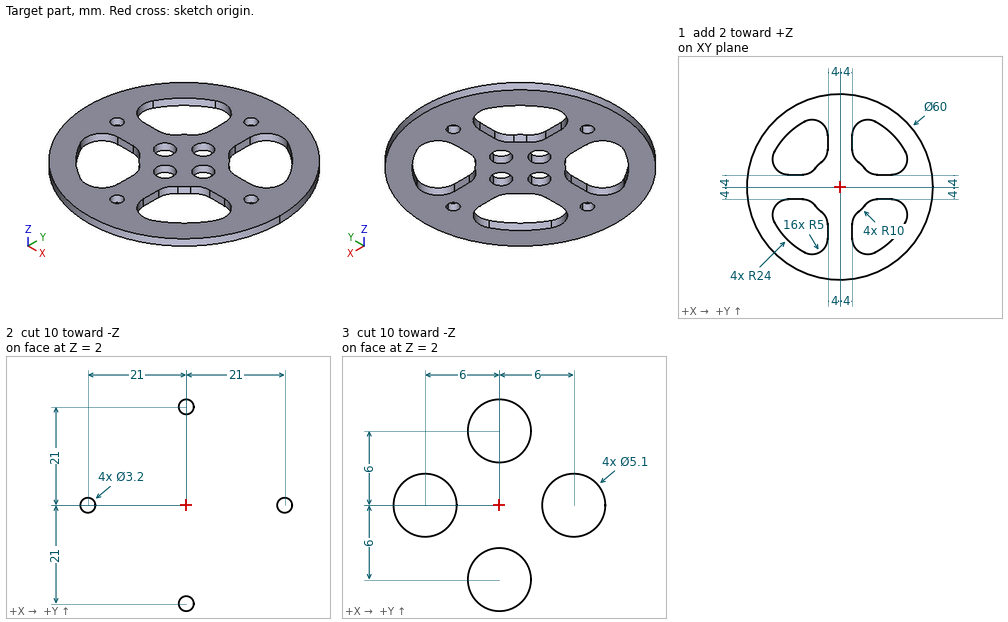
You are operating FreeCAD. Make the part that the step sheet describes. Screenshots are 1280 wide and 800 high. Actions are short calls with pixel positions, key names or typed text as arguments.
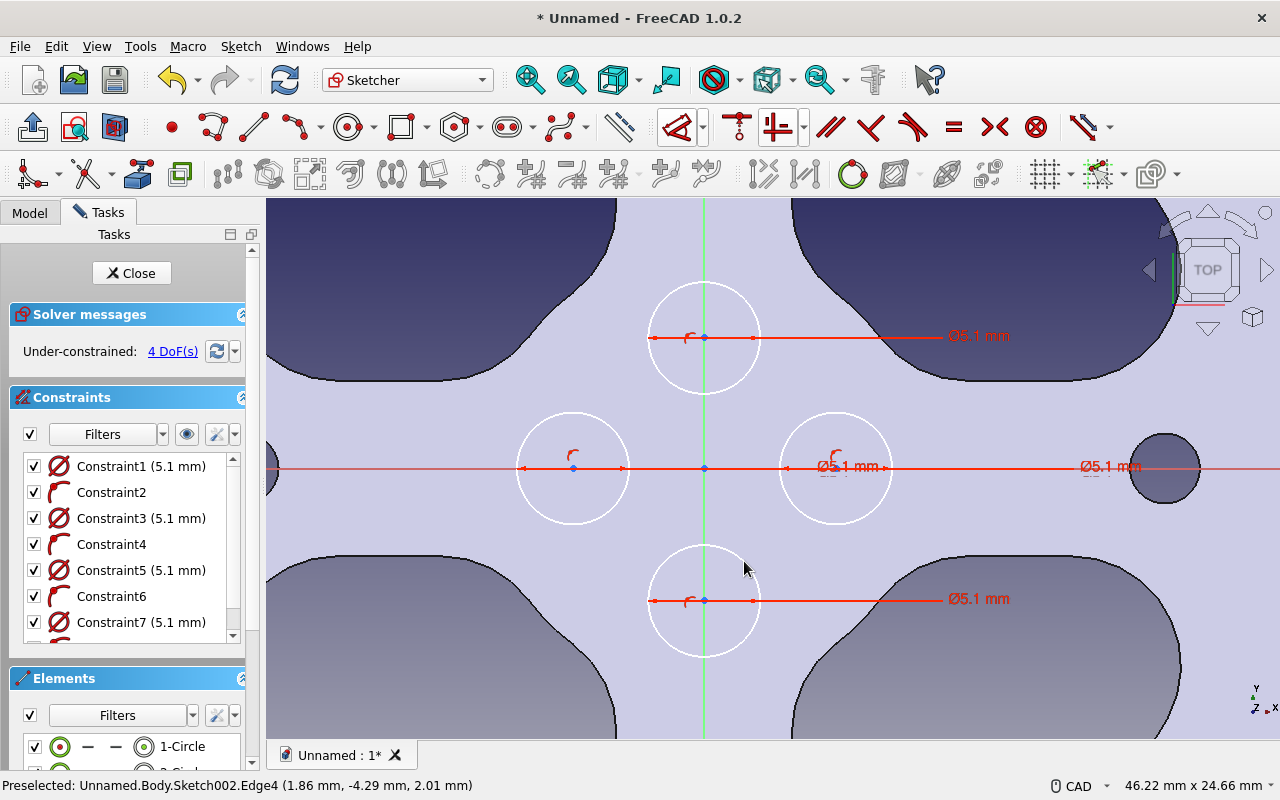
click(704, 338)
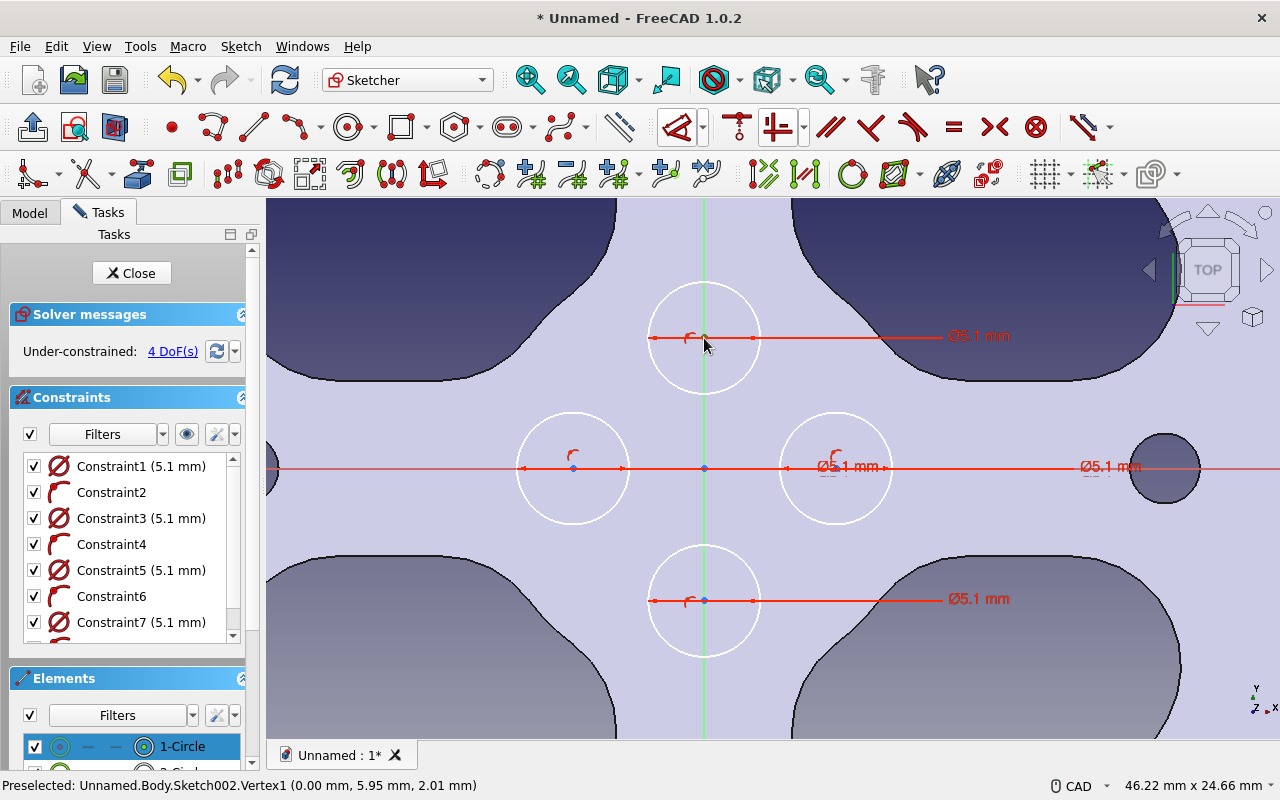
key(i)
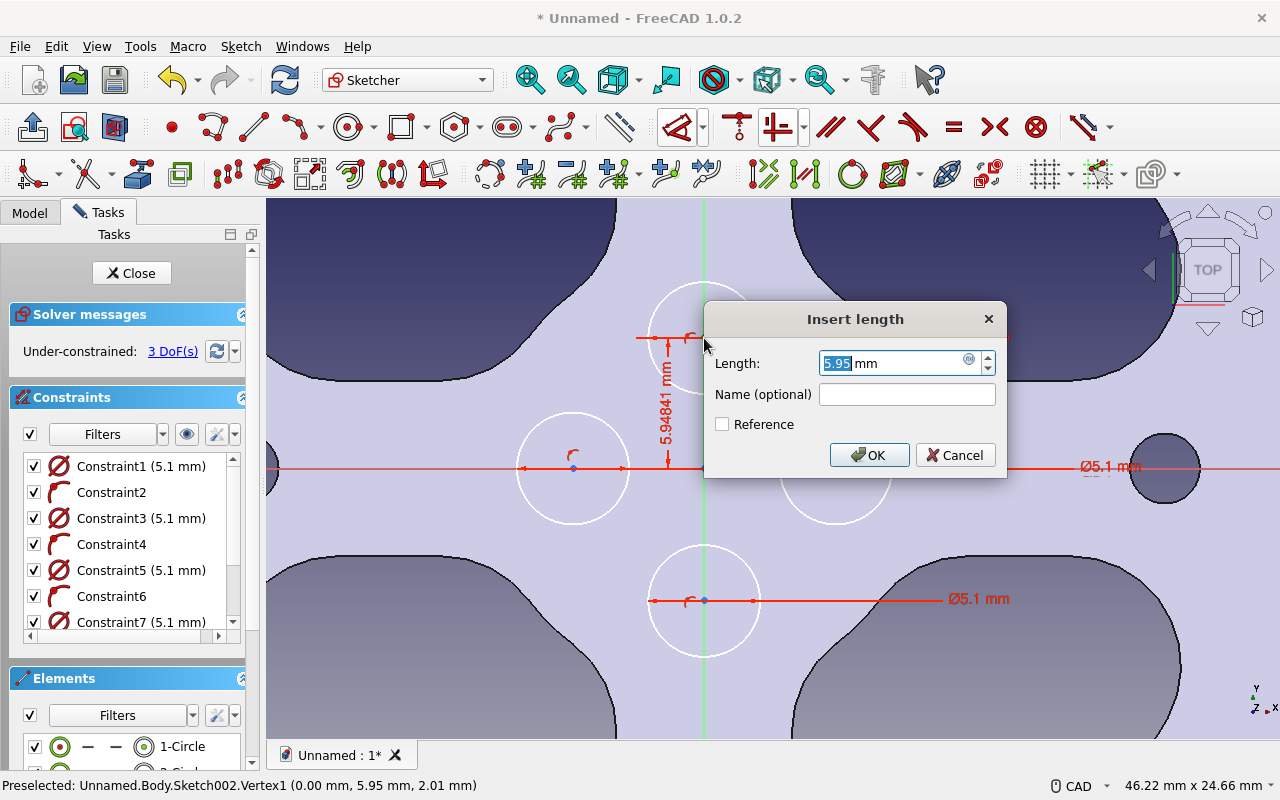
text(6)
key(Return)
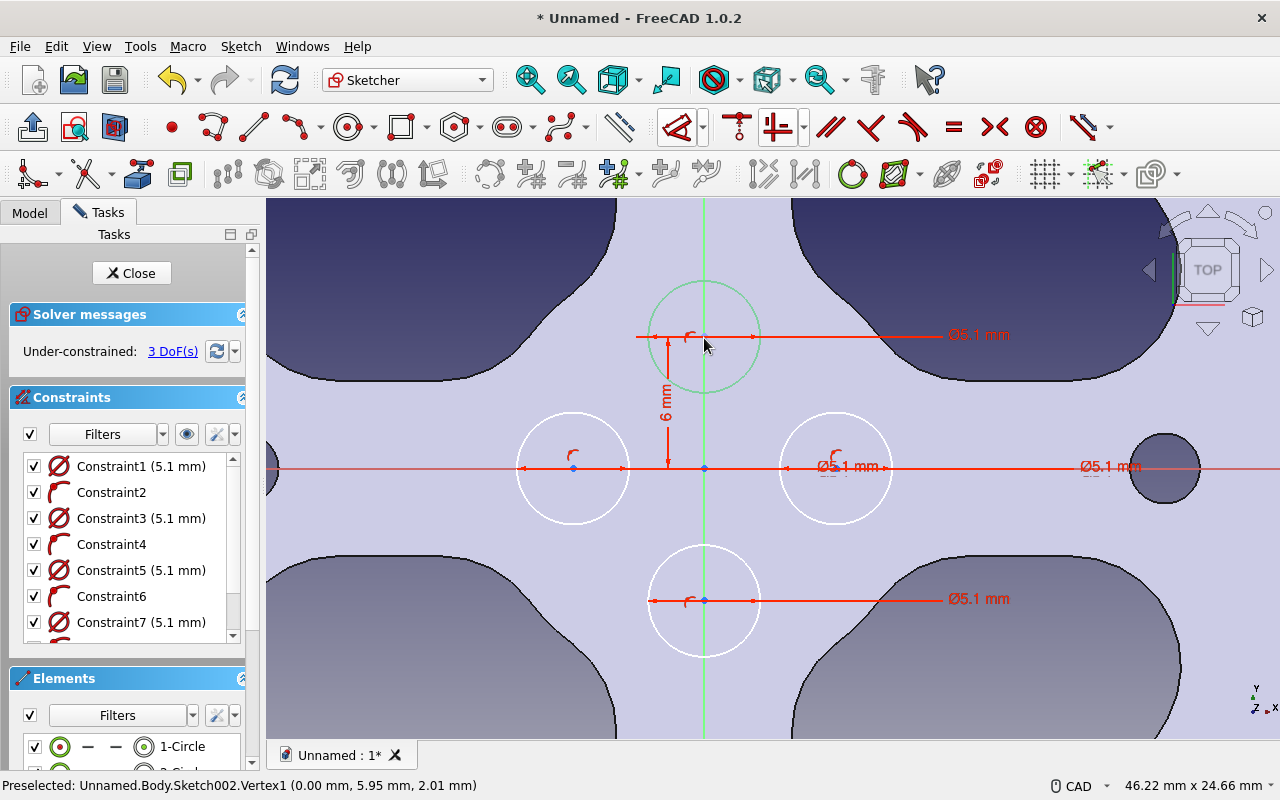
click(573, 468)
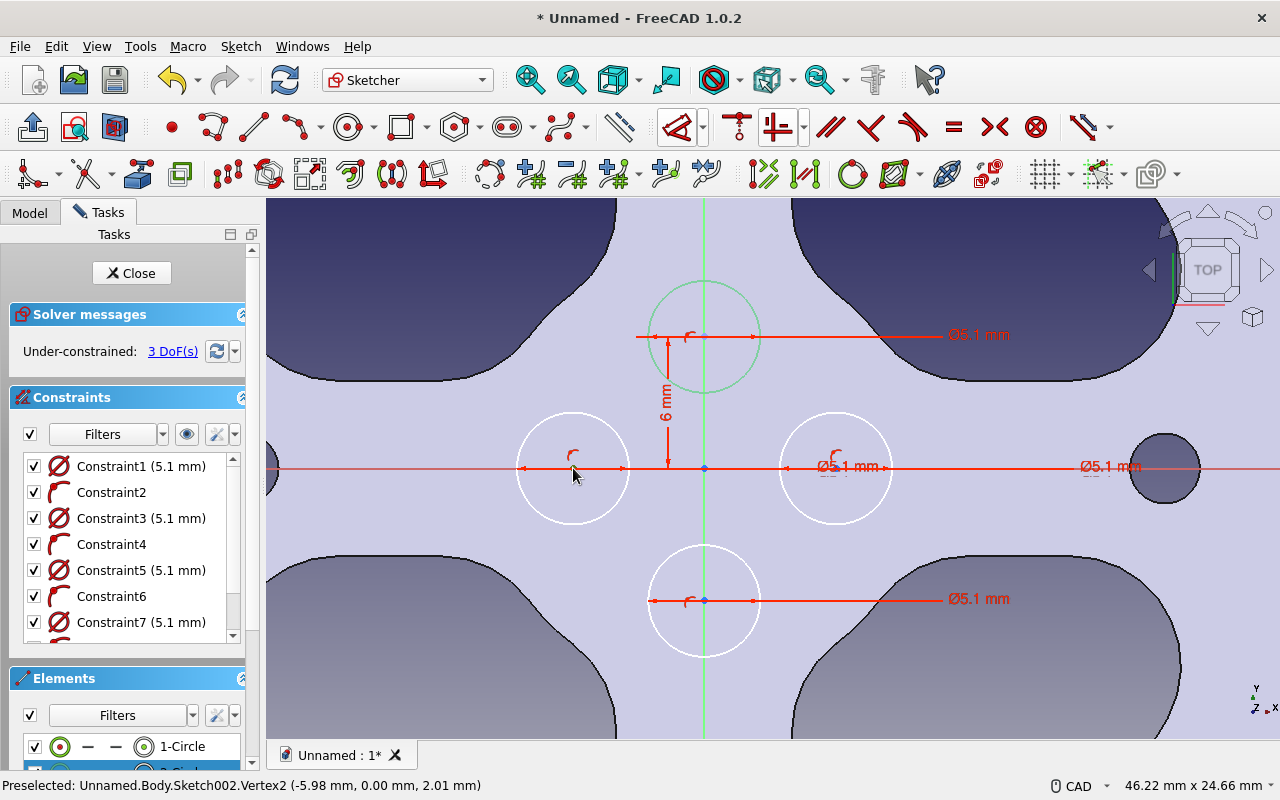
key(l)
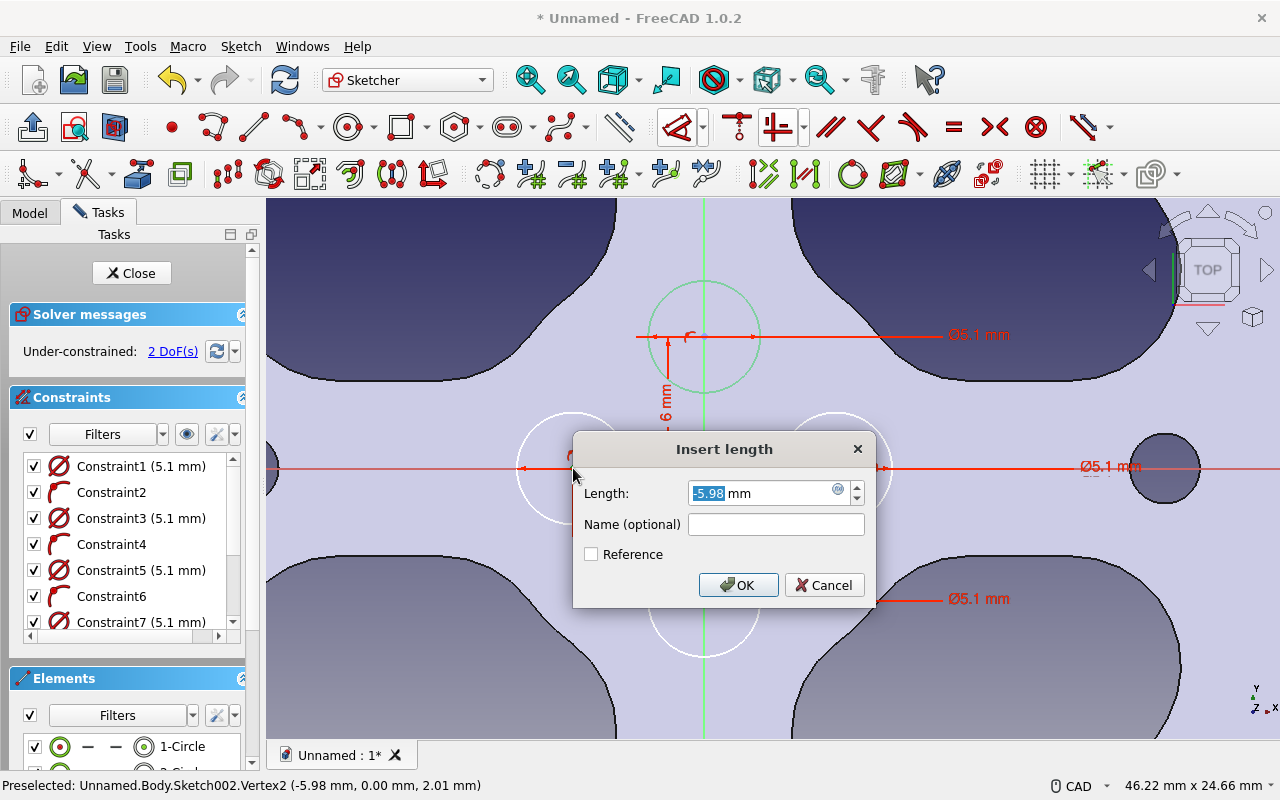
text(-6)
key(Return)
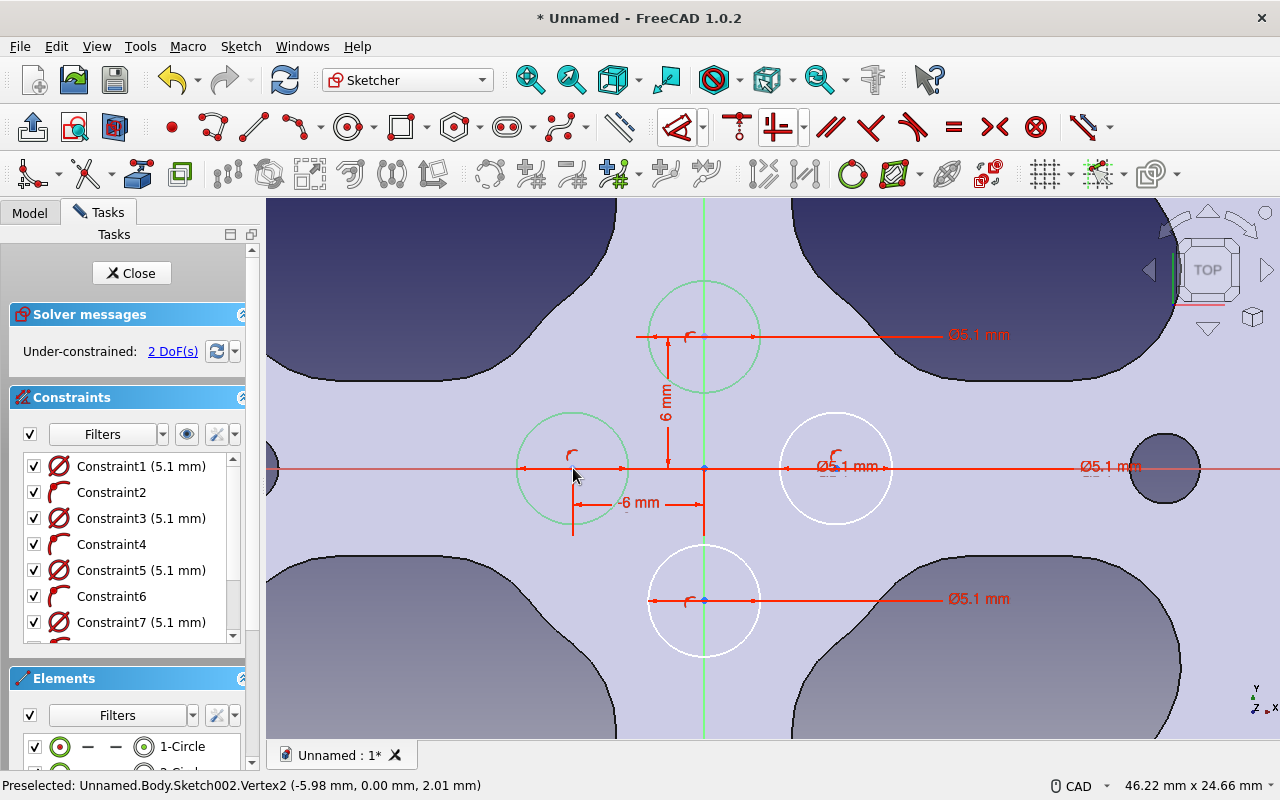
click(836, 468)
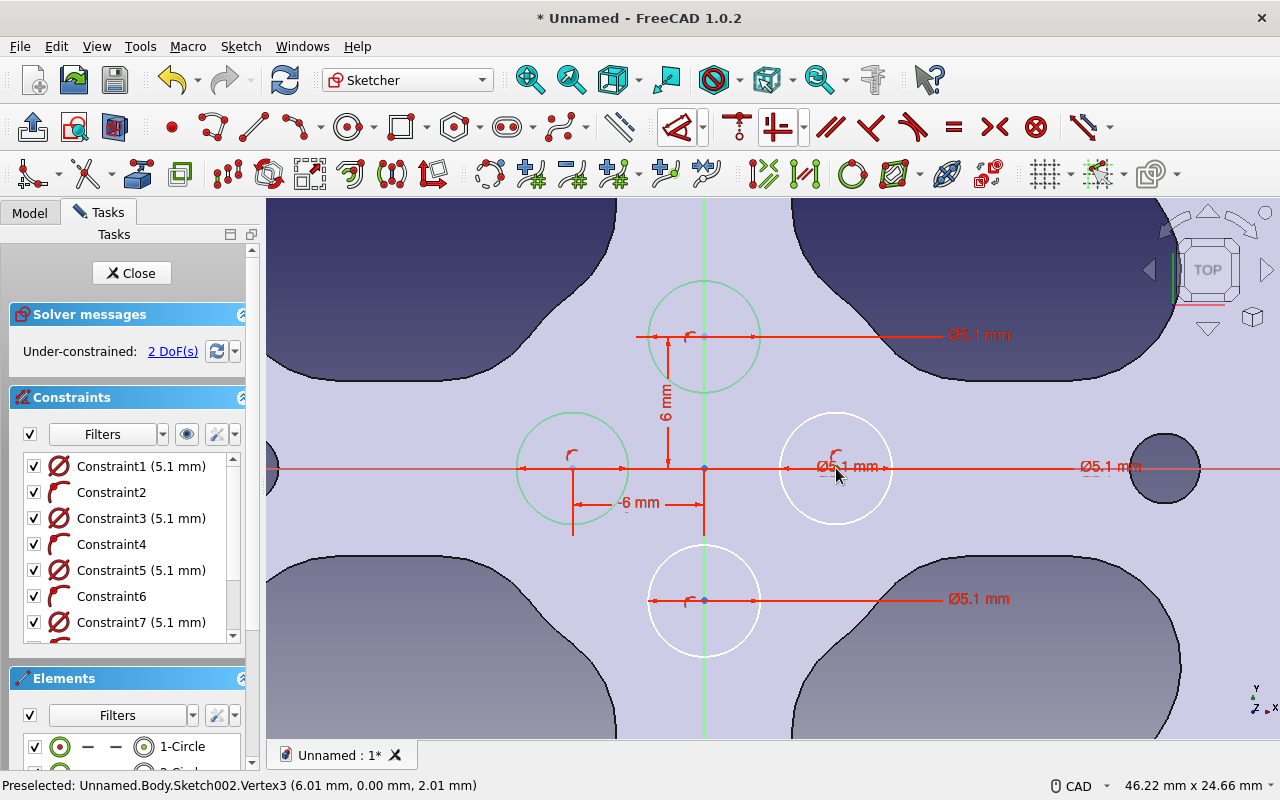
key(l)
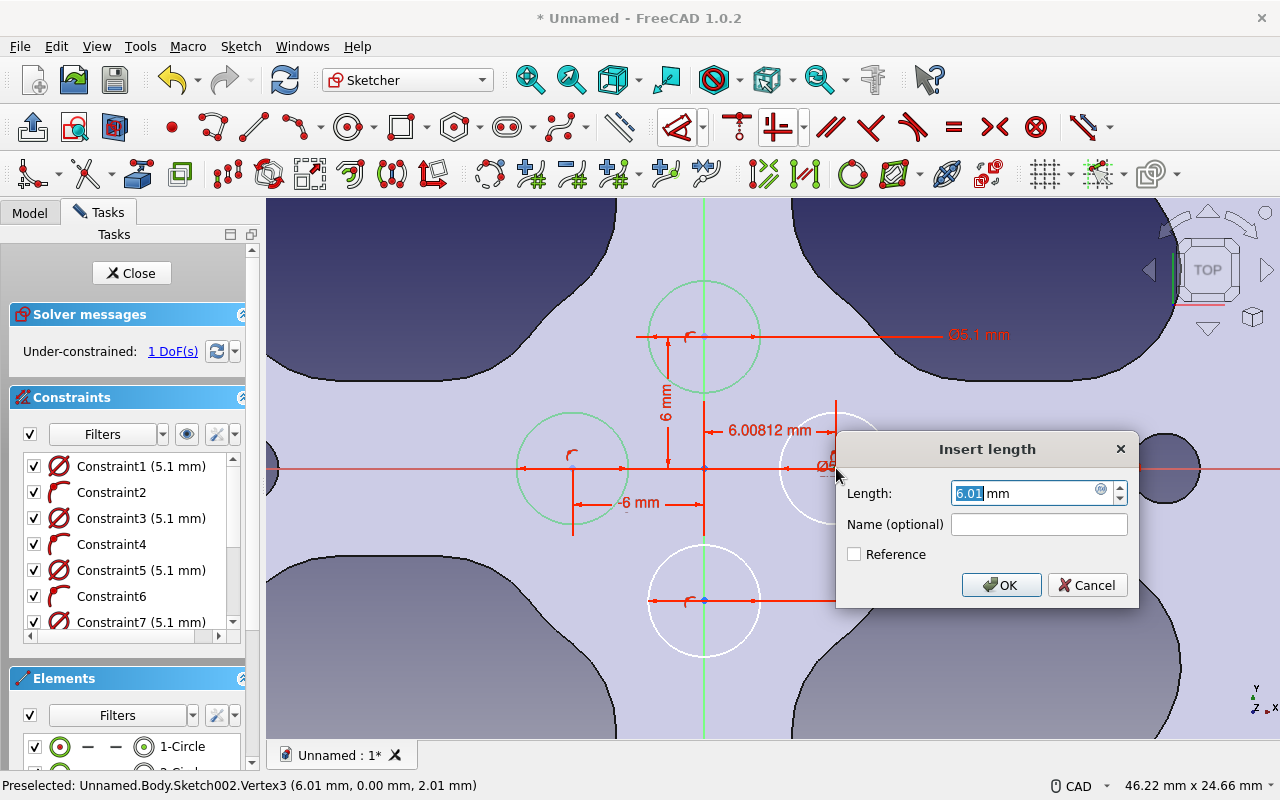
text(6)
key(Return)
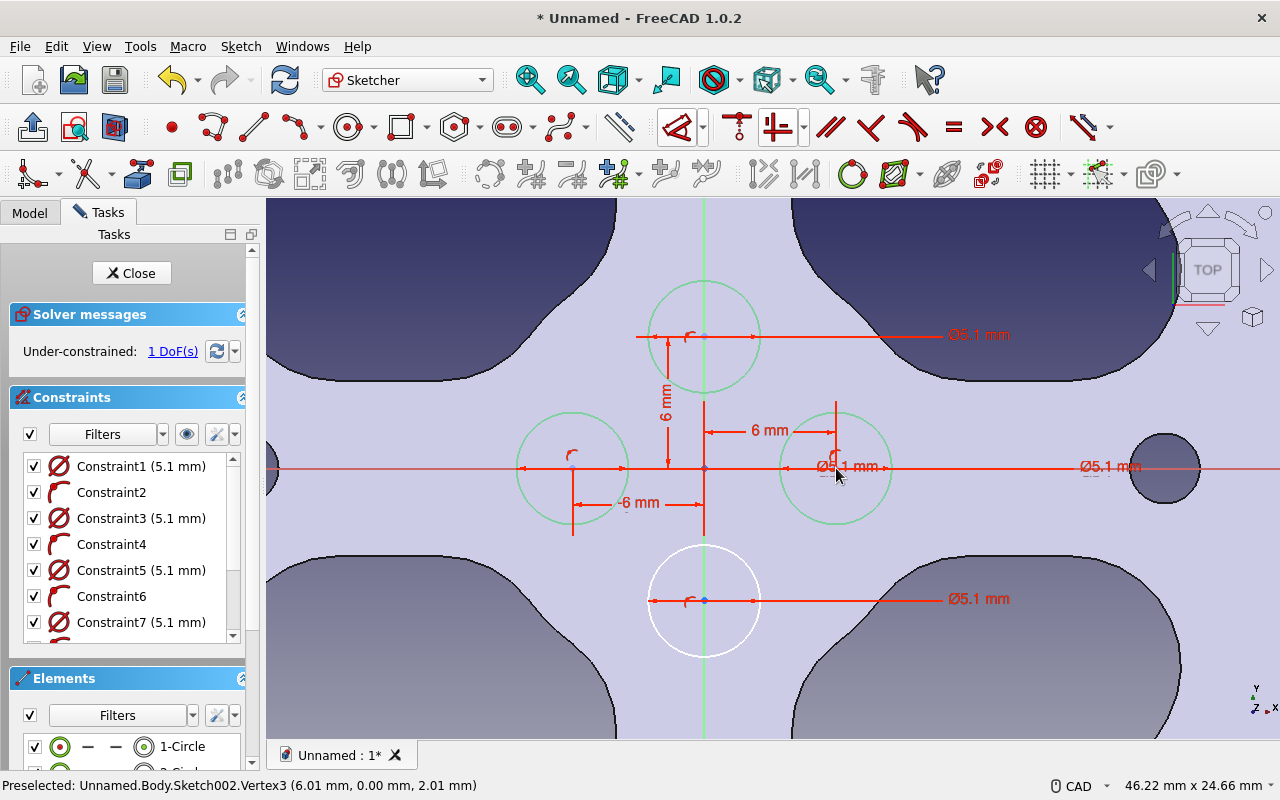
click(704, 601)